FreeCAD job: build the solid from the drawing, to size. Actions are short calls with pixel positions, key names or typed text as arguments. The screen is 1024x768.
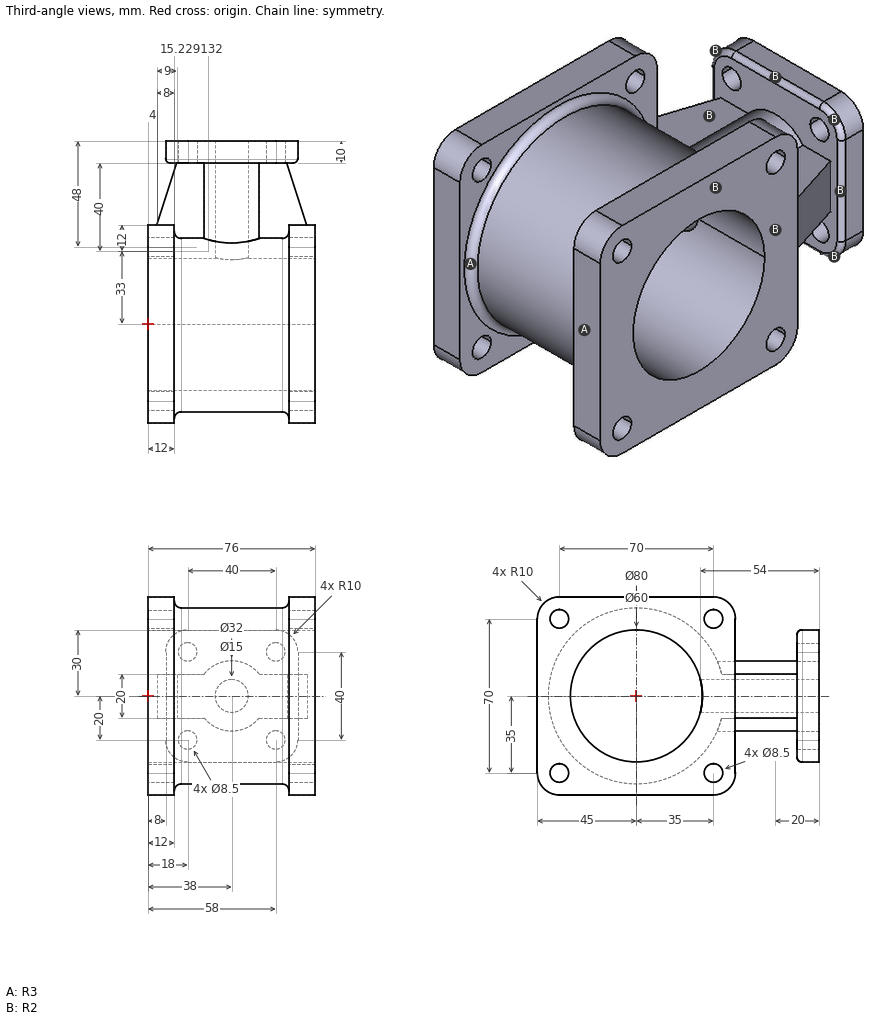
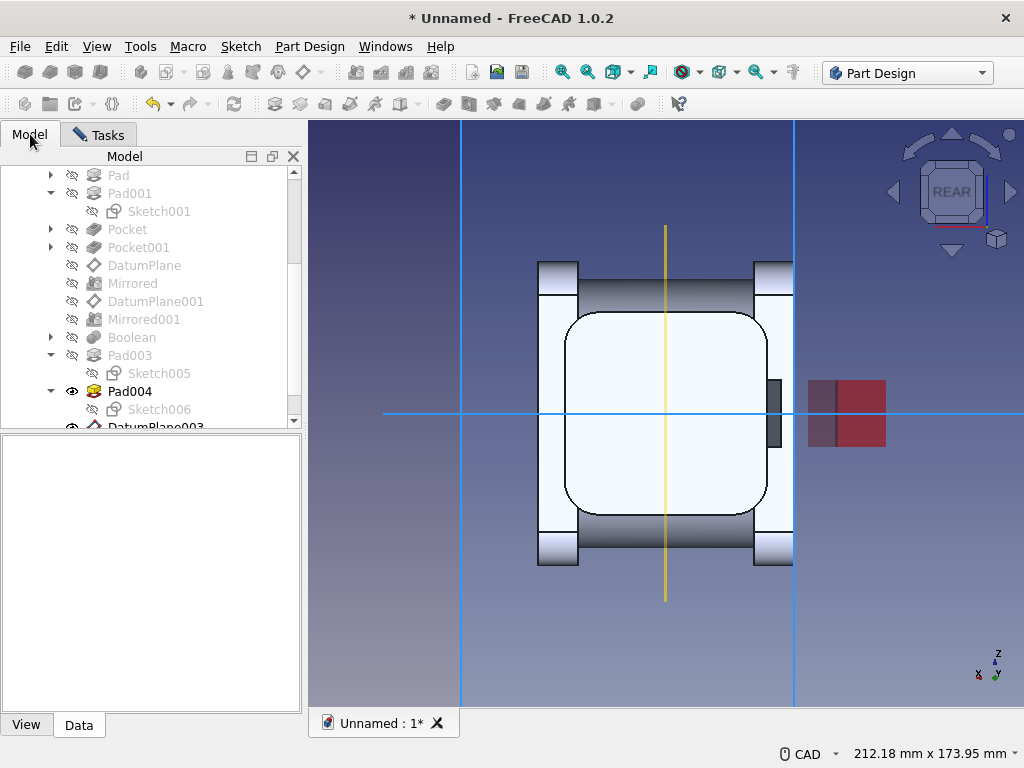
click(117, 427)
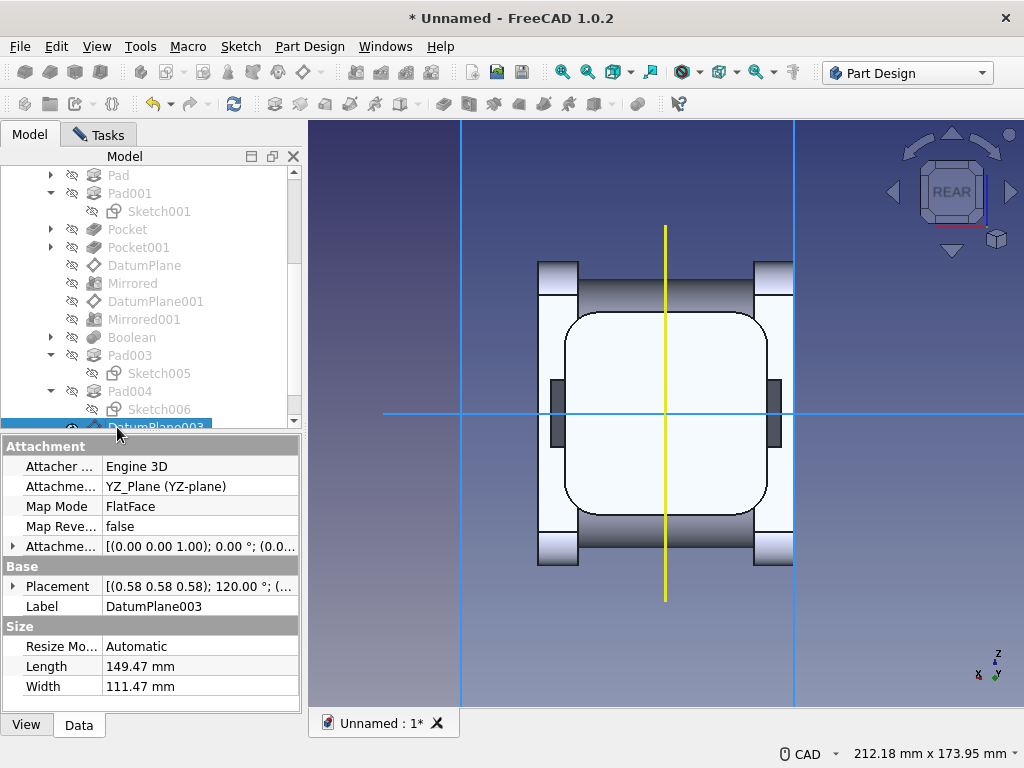
click(98, 134)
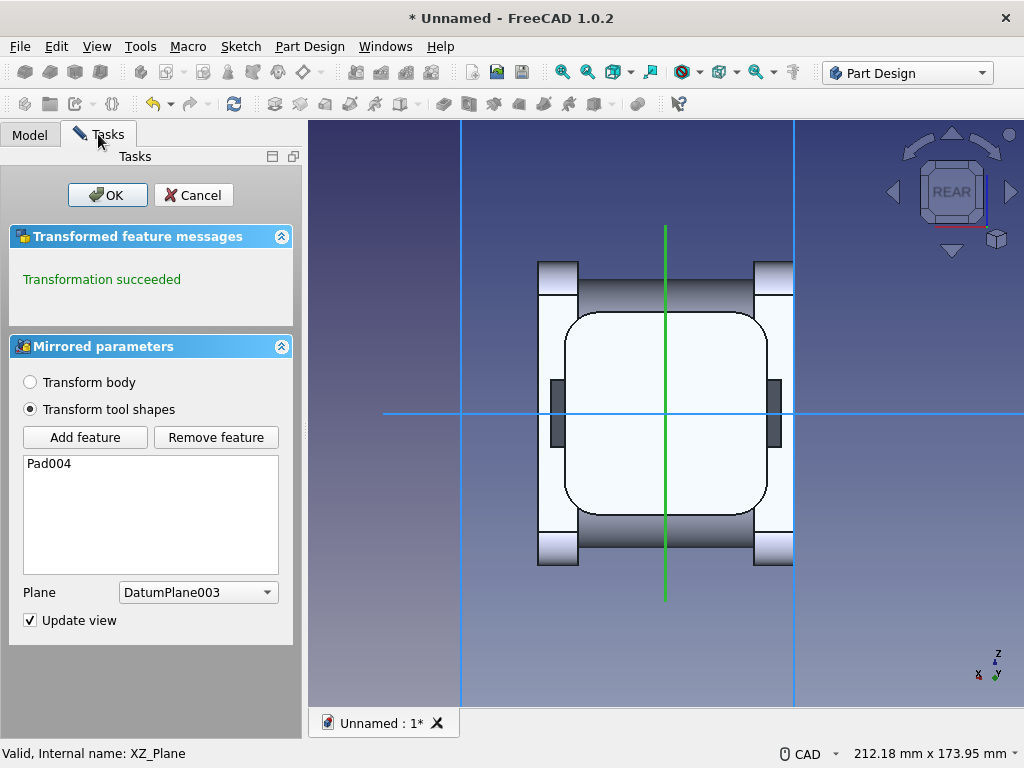
click(108, 195)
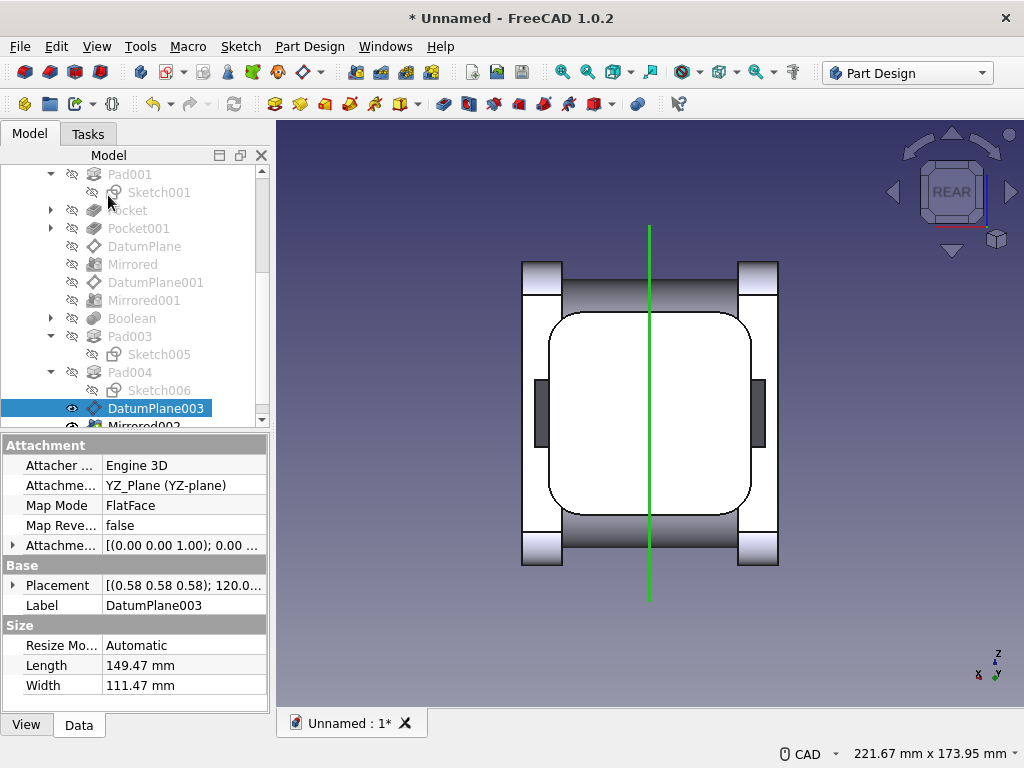
click(117, 408)
key(space)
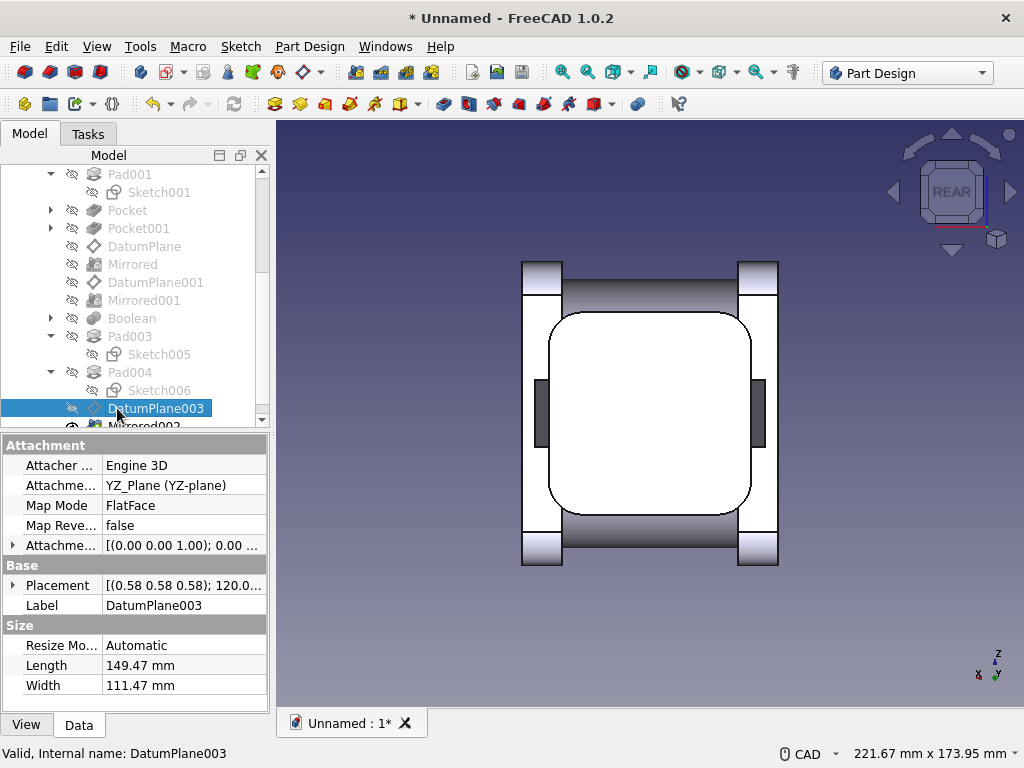
click(650, 412)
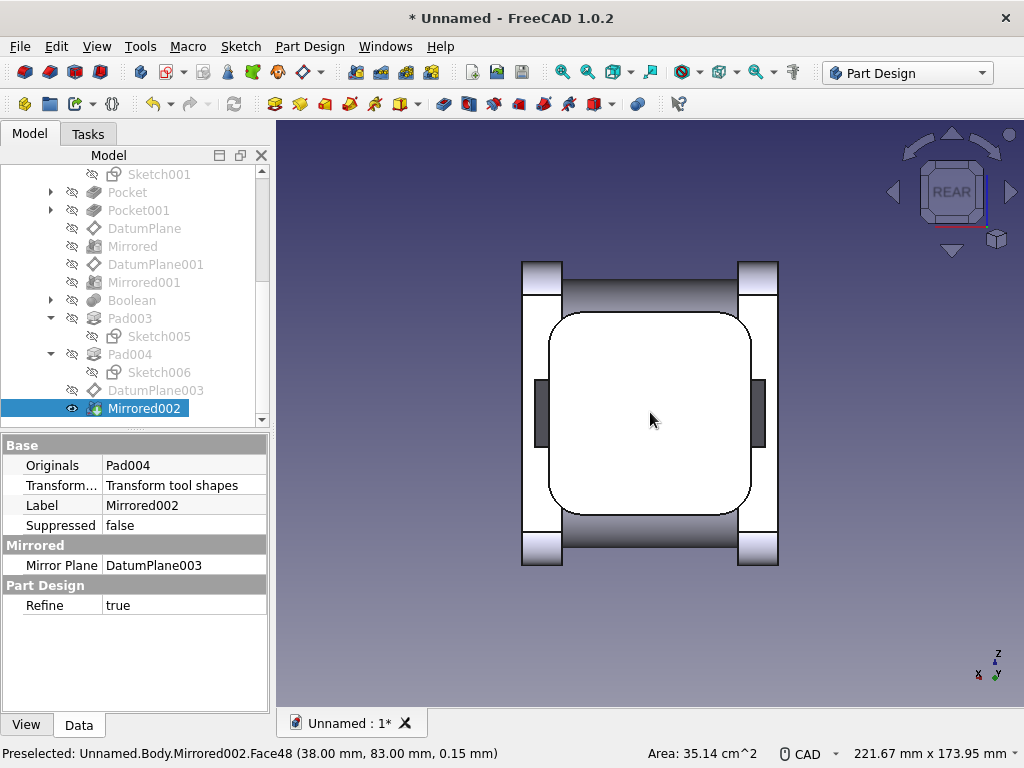
click(166, 72)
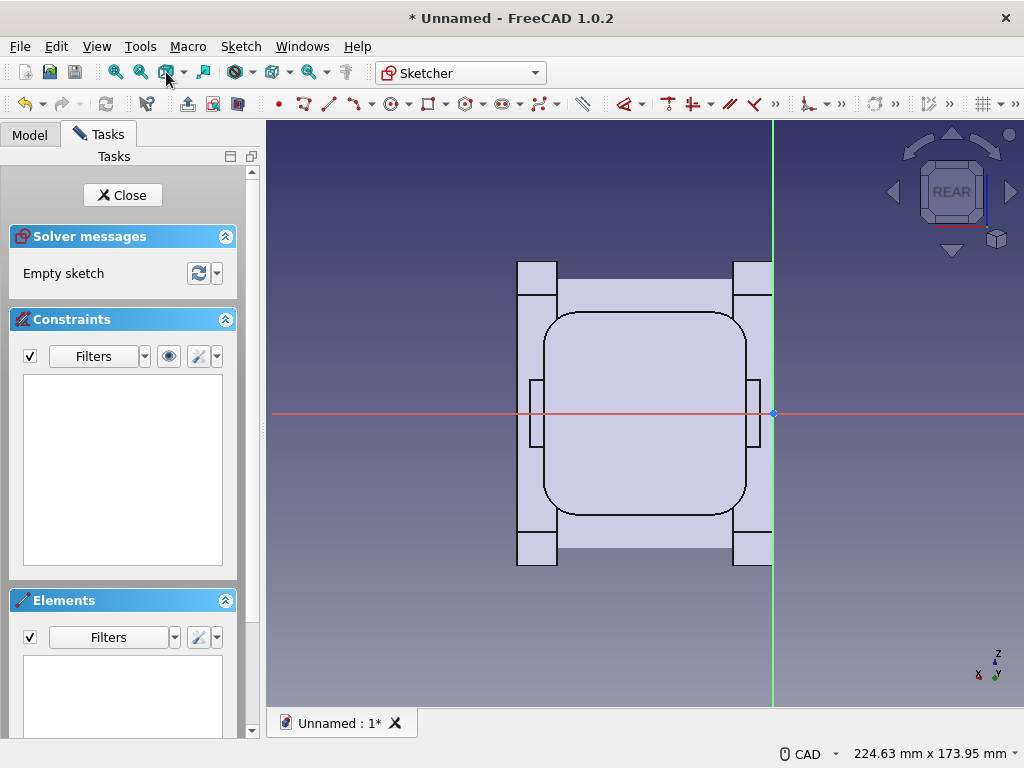
scroll(780, 414, up, 3)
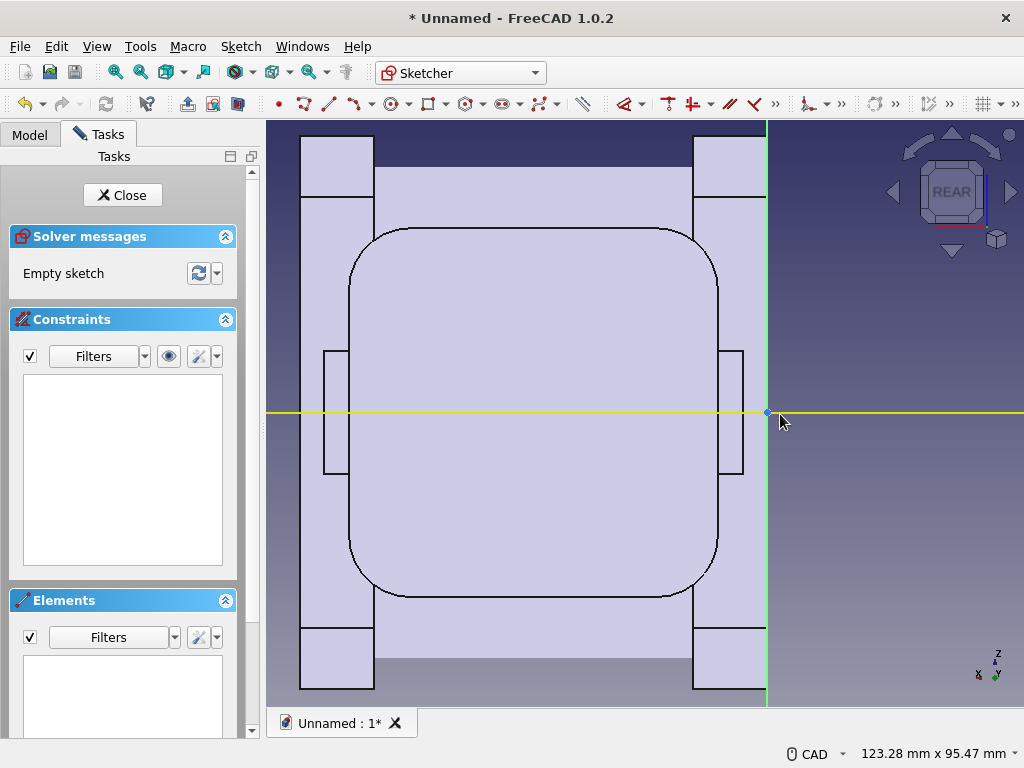
key(g)
key(c)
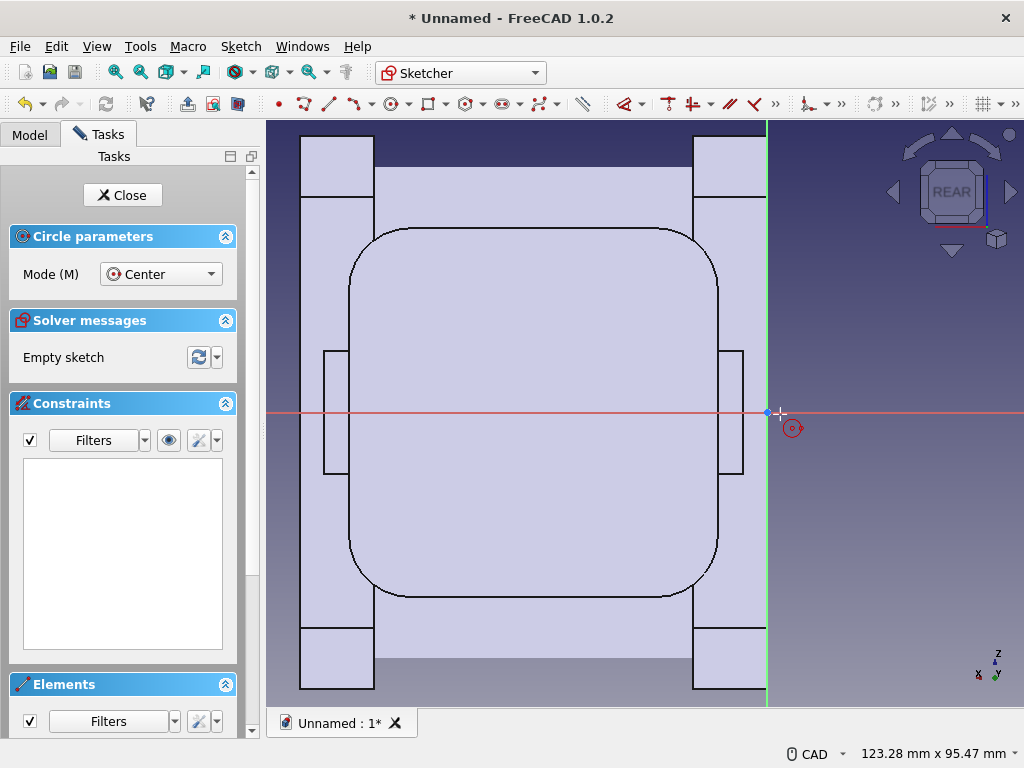
click(656, 536)
click(675, 517)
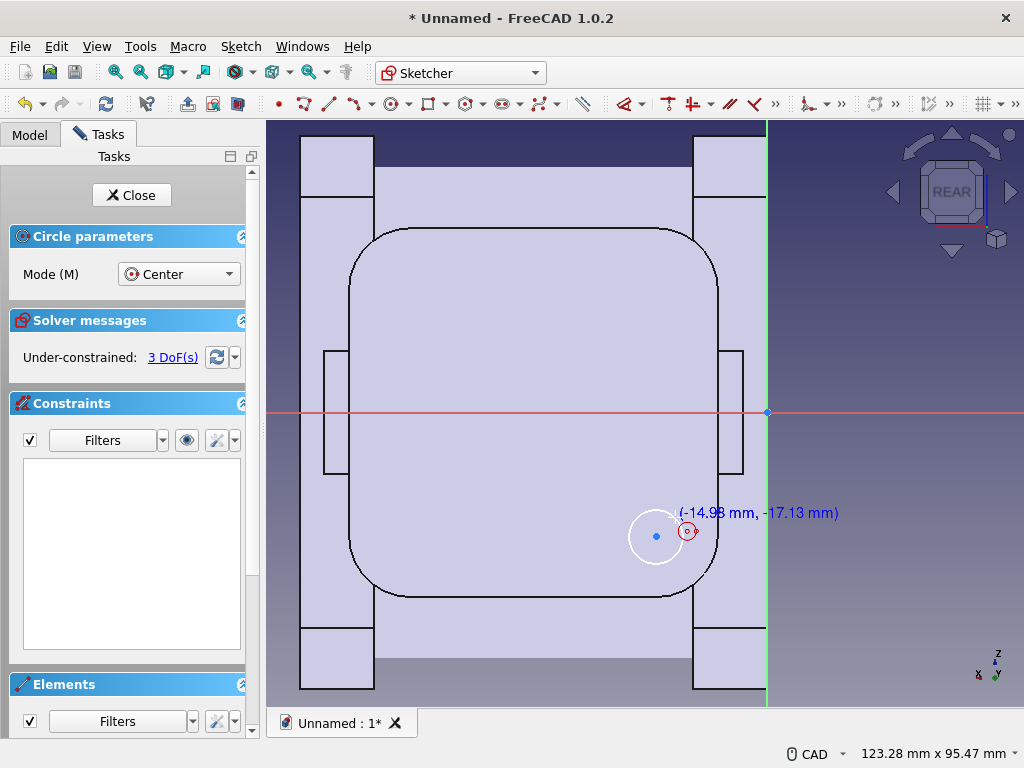
click(410, 536)
click(429, 517)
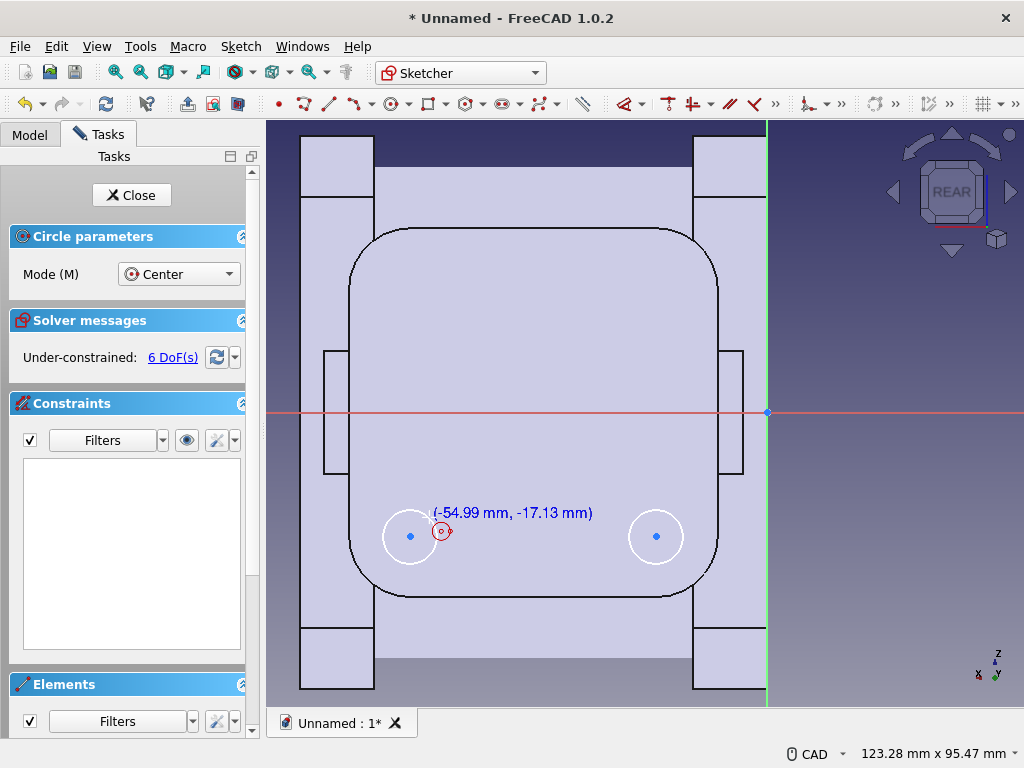
click(656, 290)
click(675, 271)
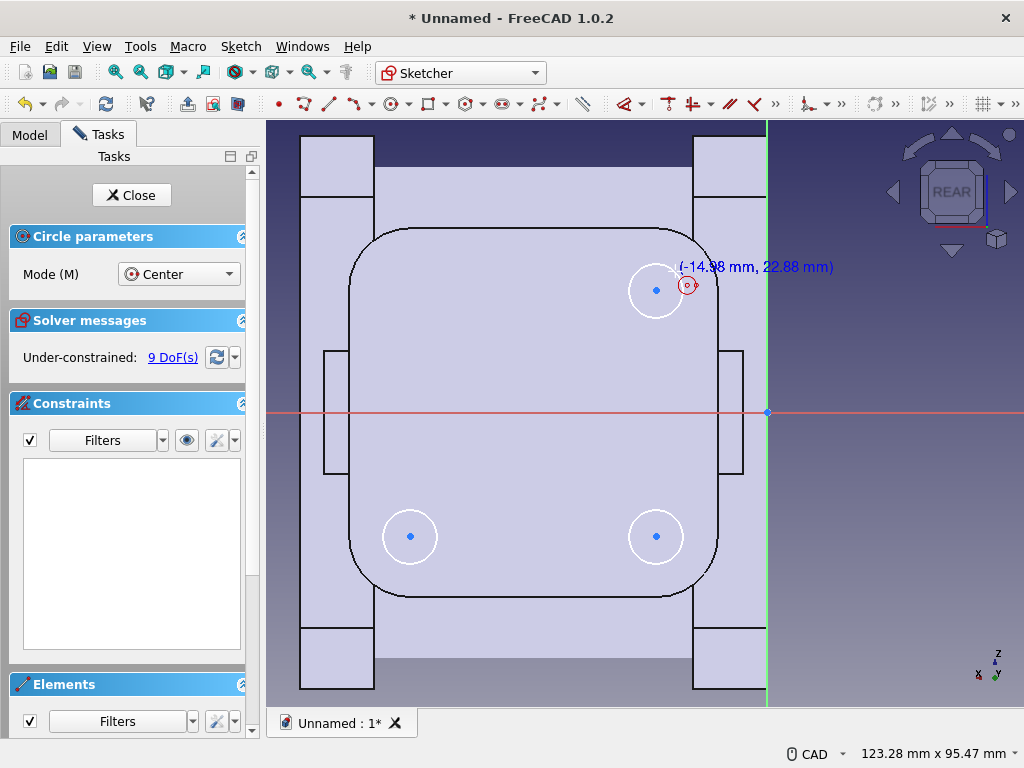
click(410, 290)
click(429, 271)
key(Escape)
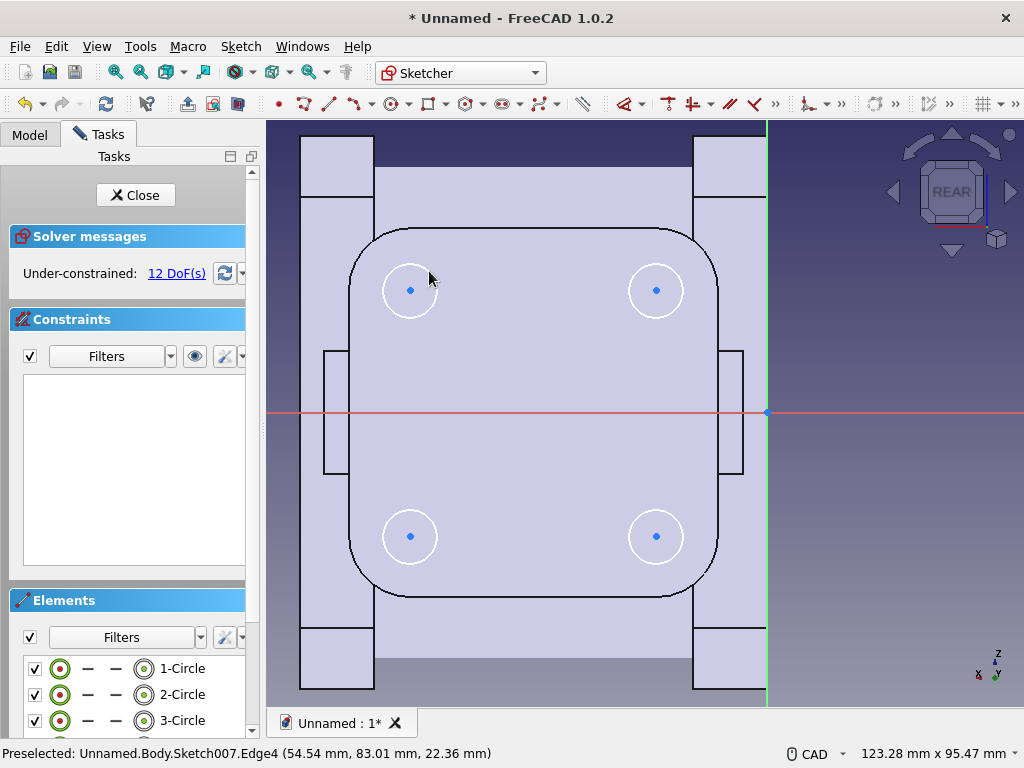
click(675, 518)